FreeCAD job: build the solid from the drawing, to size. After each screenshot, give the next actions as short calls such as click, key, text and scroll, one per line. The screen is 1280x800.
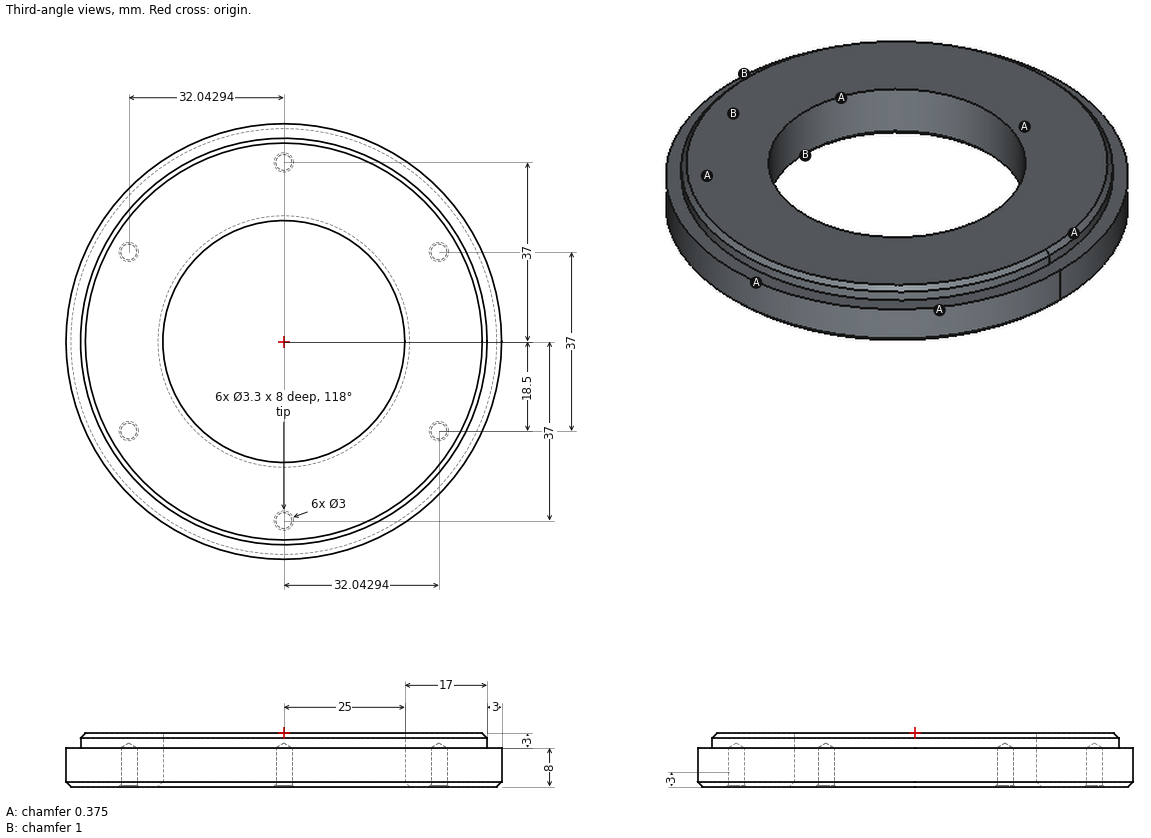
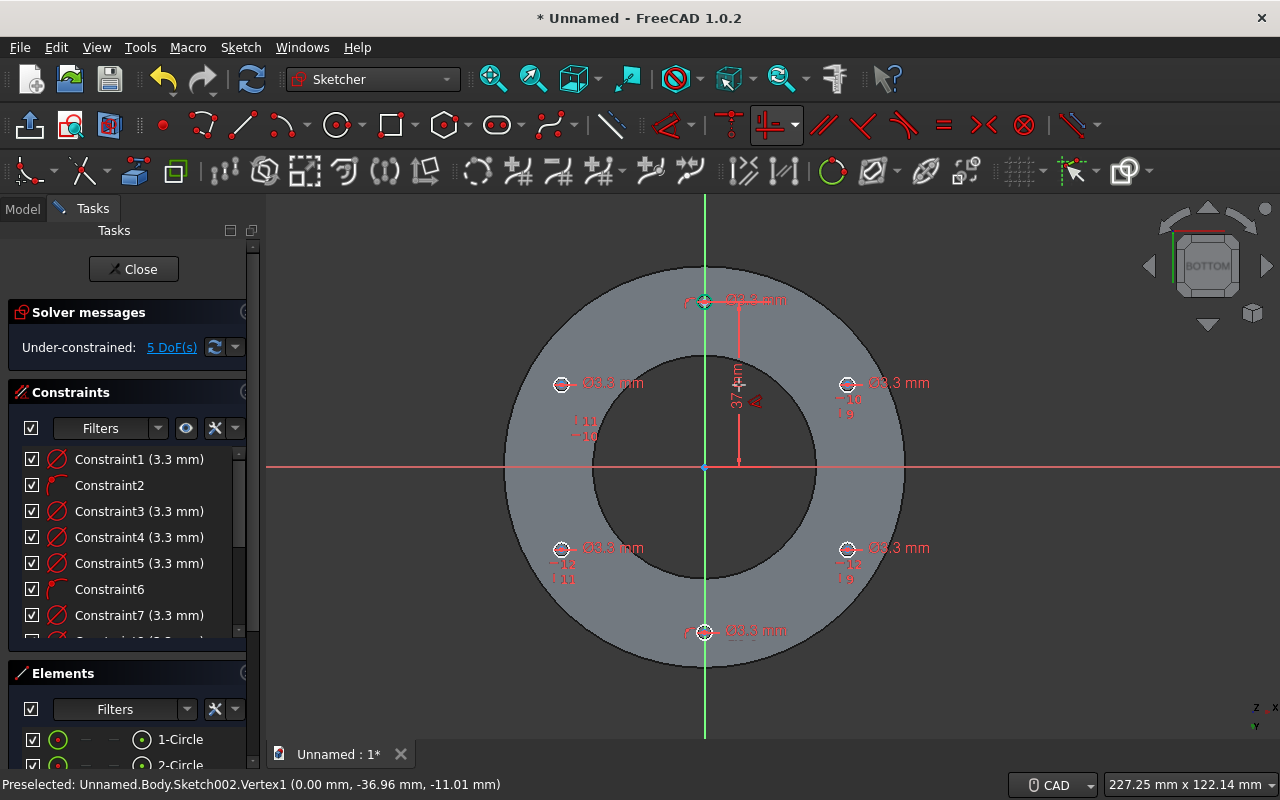
click(705, 633)
click(739, 550)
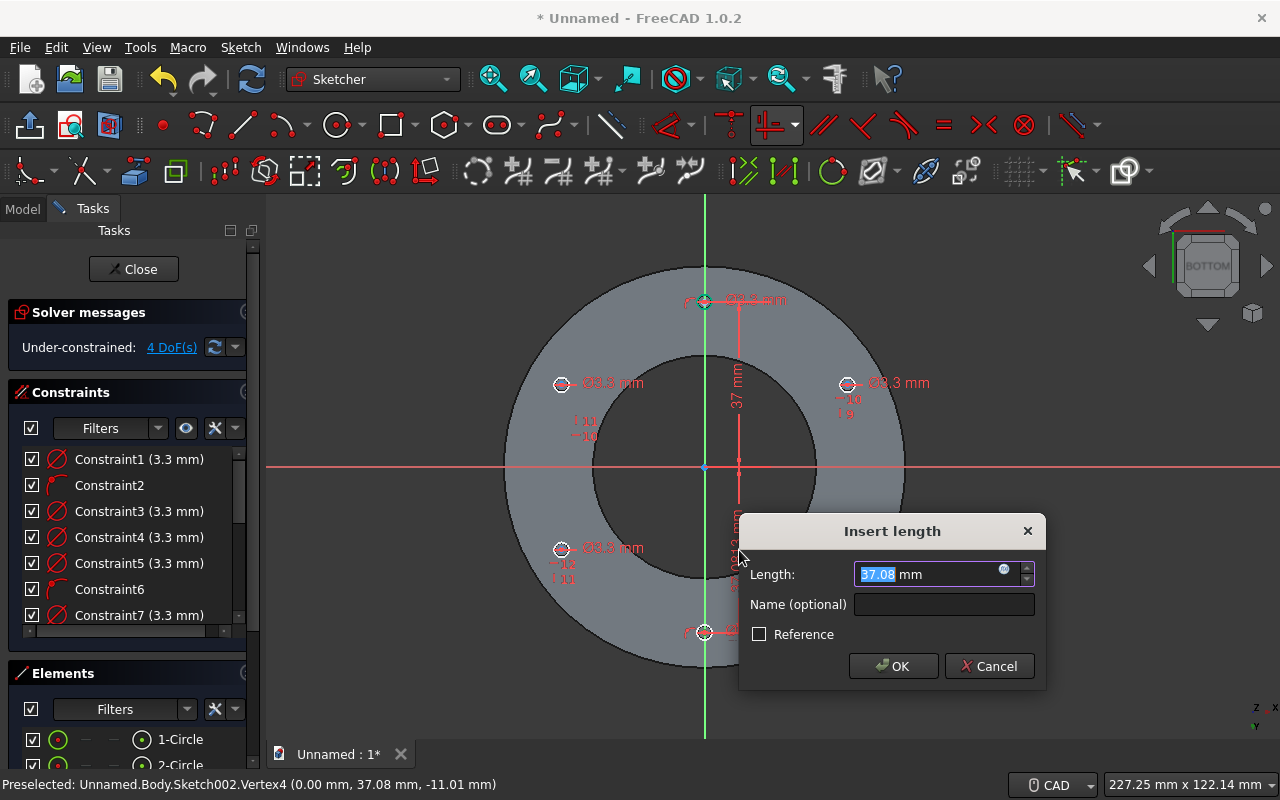
text(37)
key(Return)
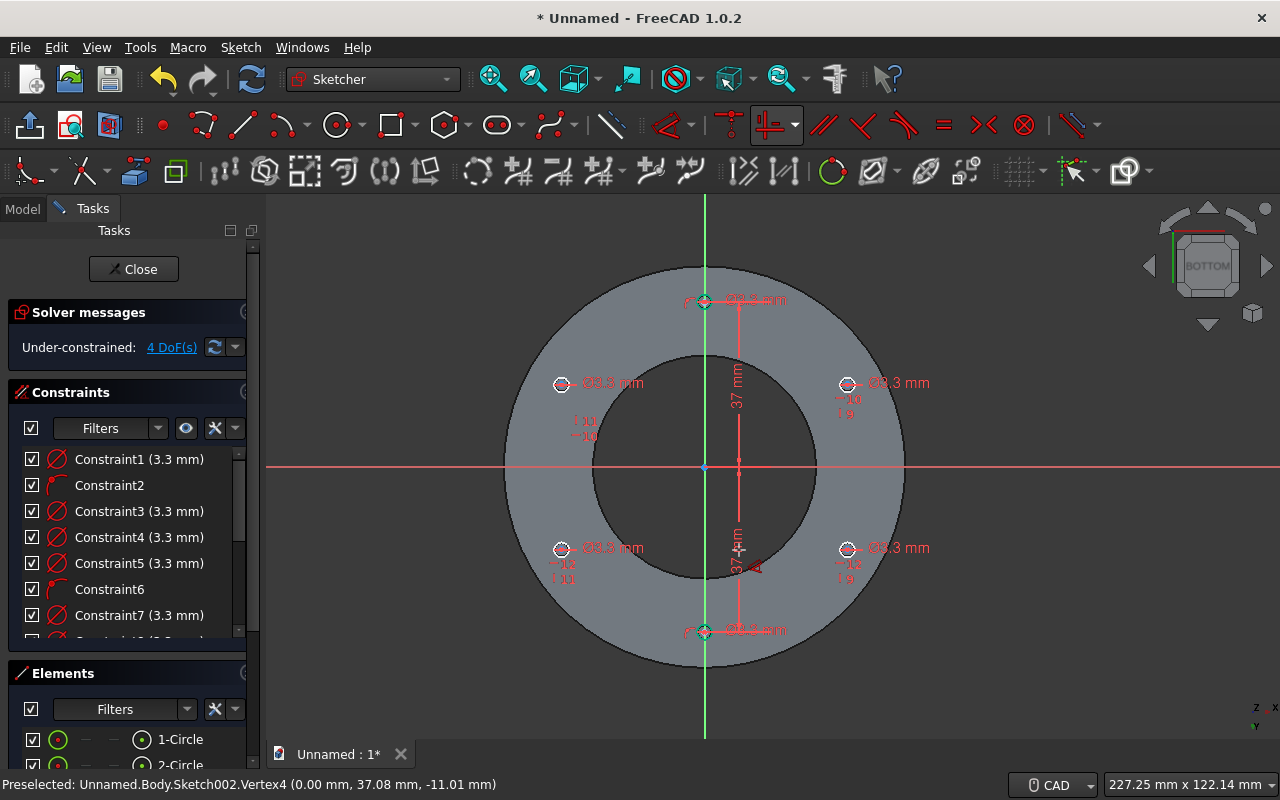
click(847, 385)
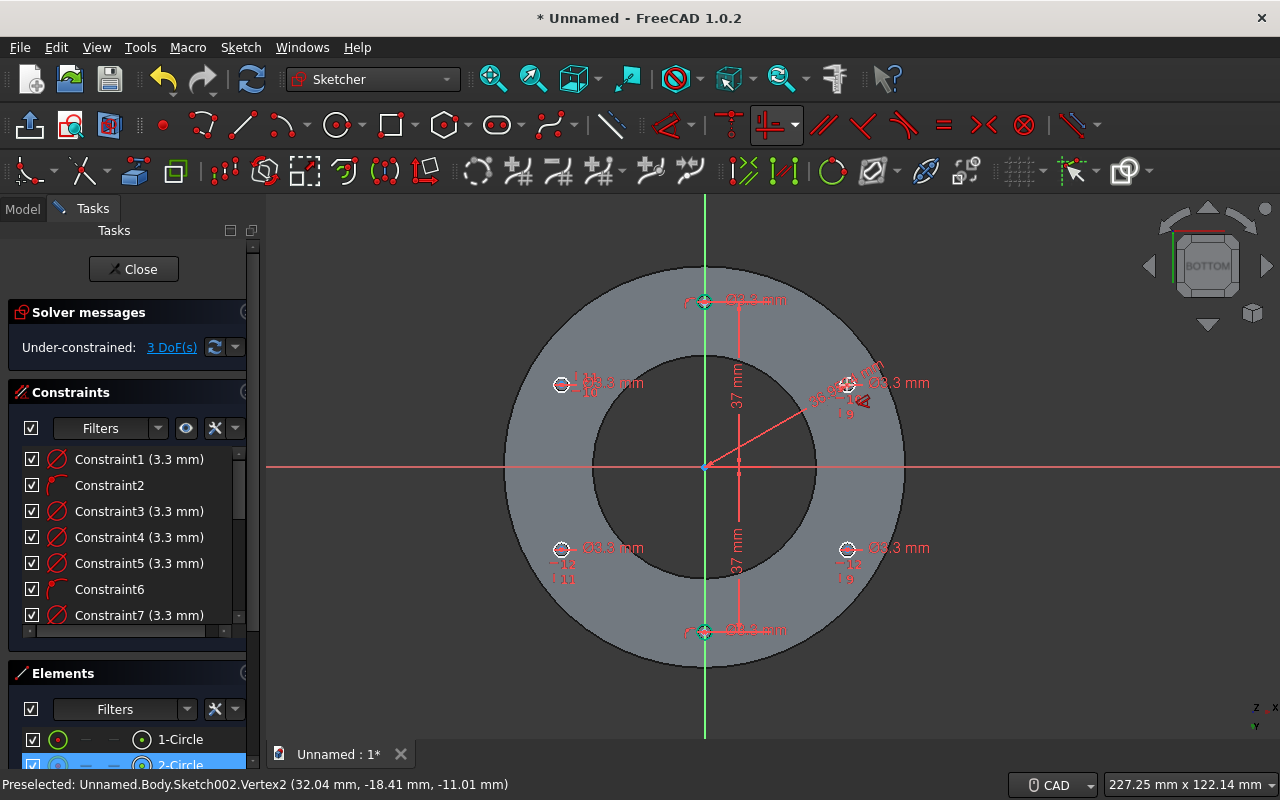
click(847, 550)
click(881, 429)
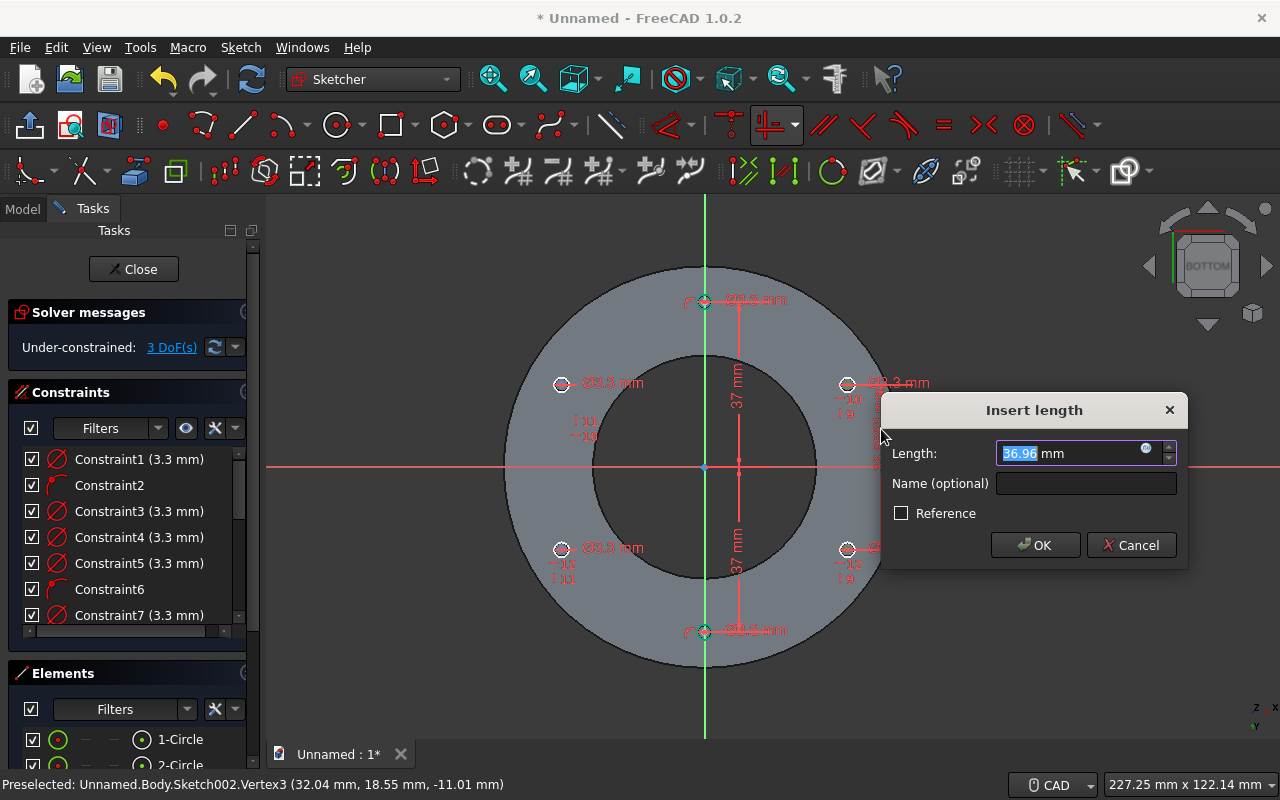
text(37)
key(Return)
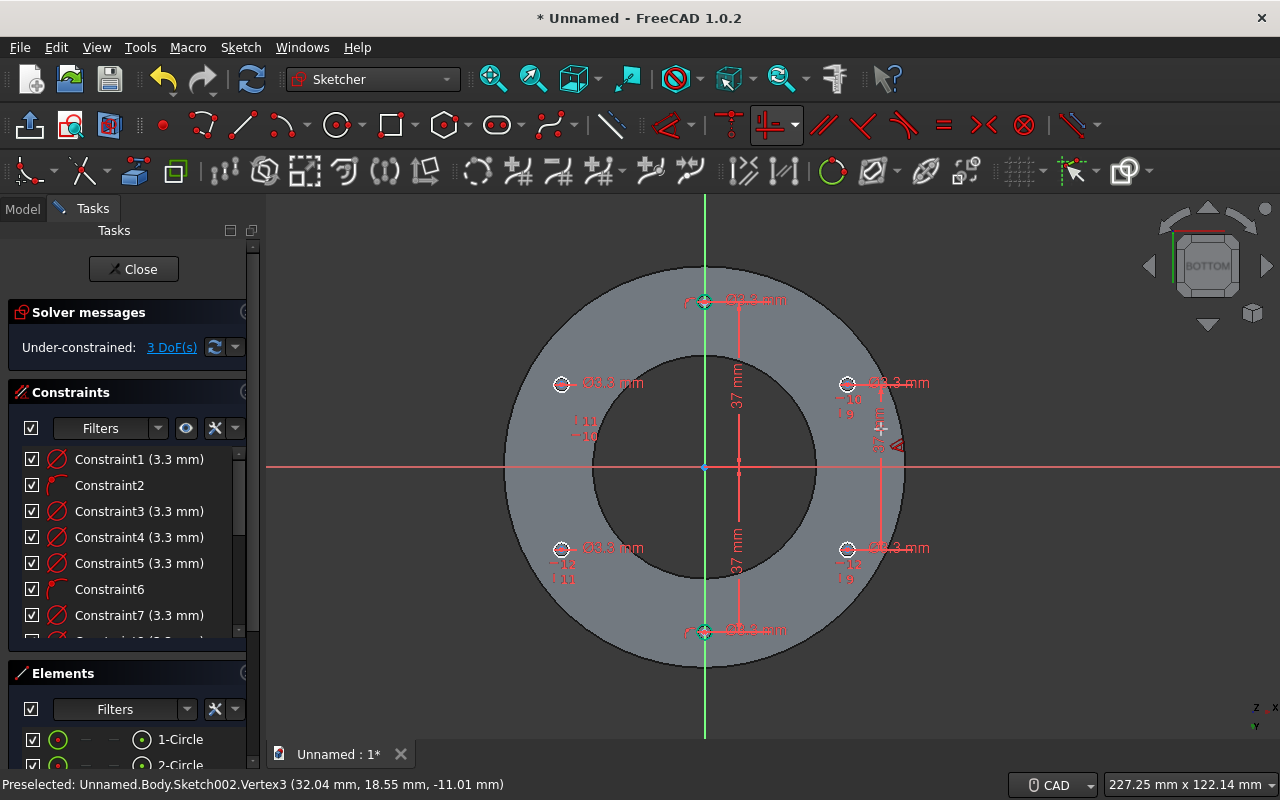
click(847, 385)
click(881, 407)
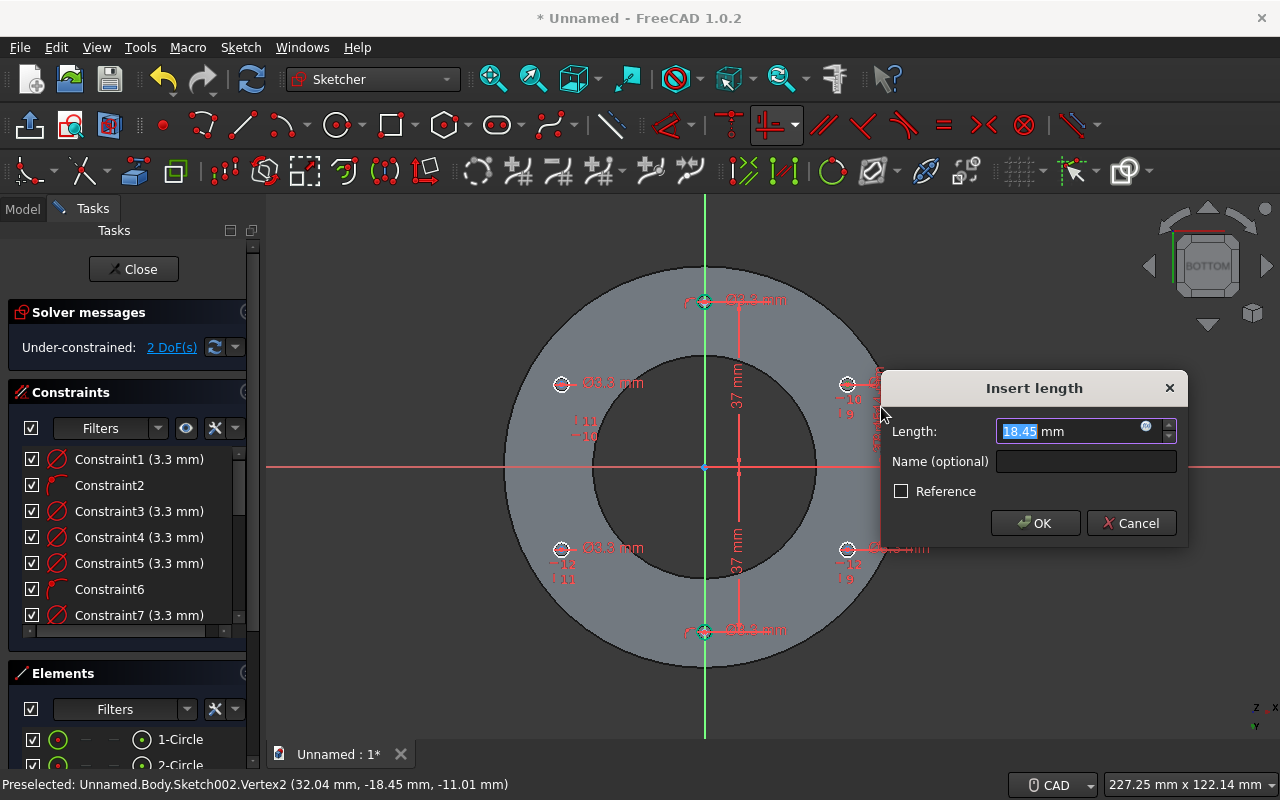
text(18.5)
key(Return)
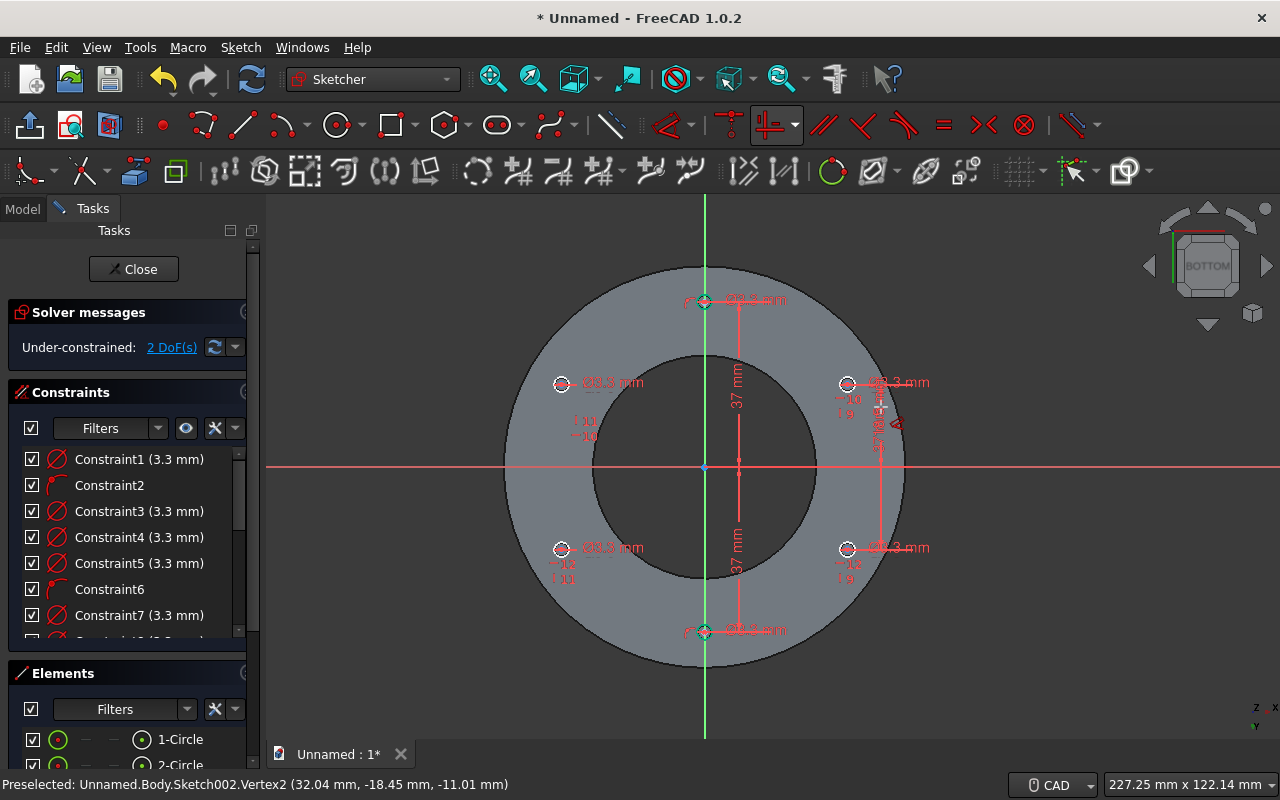
click(847, 385)
click(776, 351)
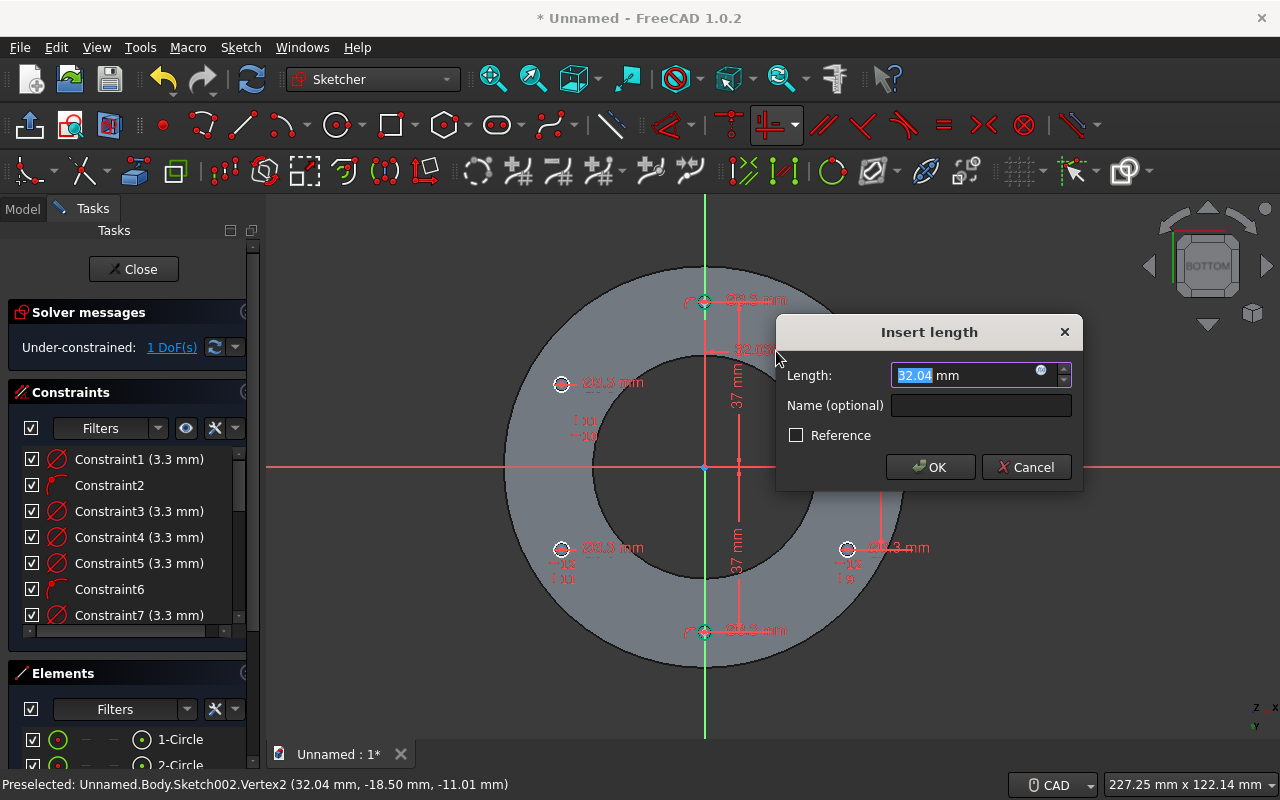
text(32.04294)
key(Return)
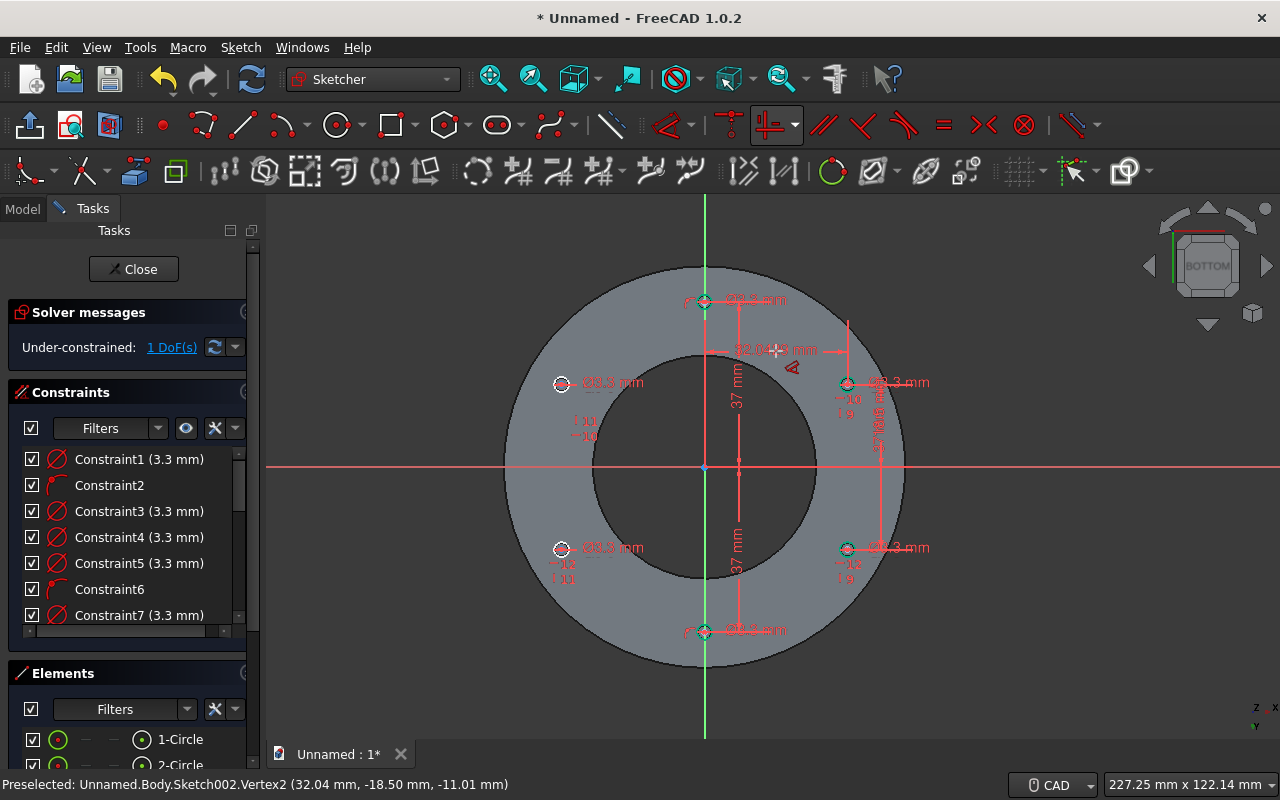
click(562, 385)
click(633, 351)